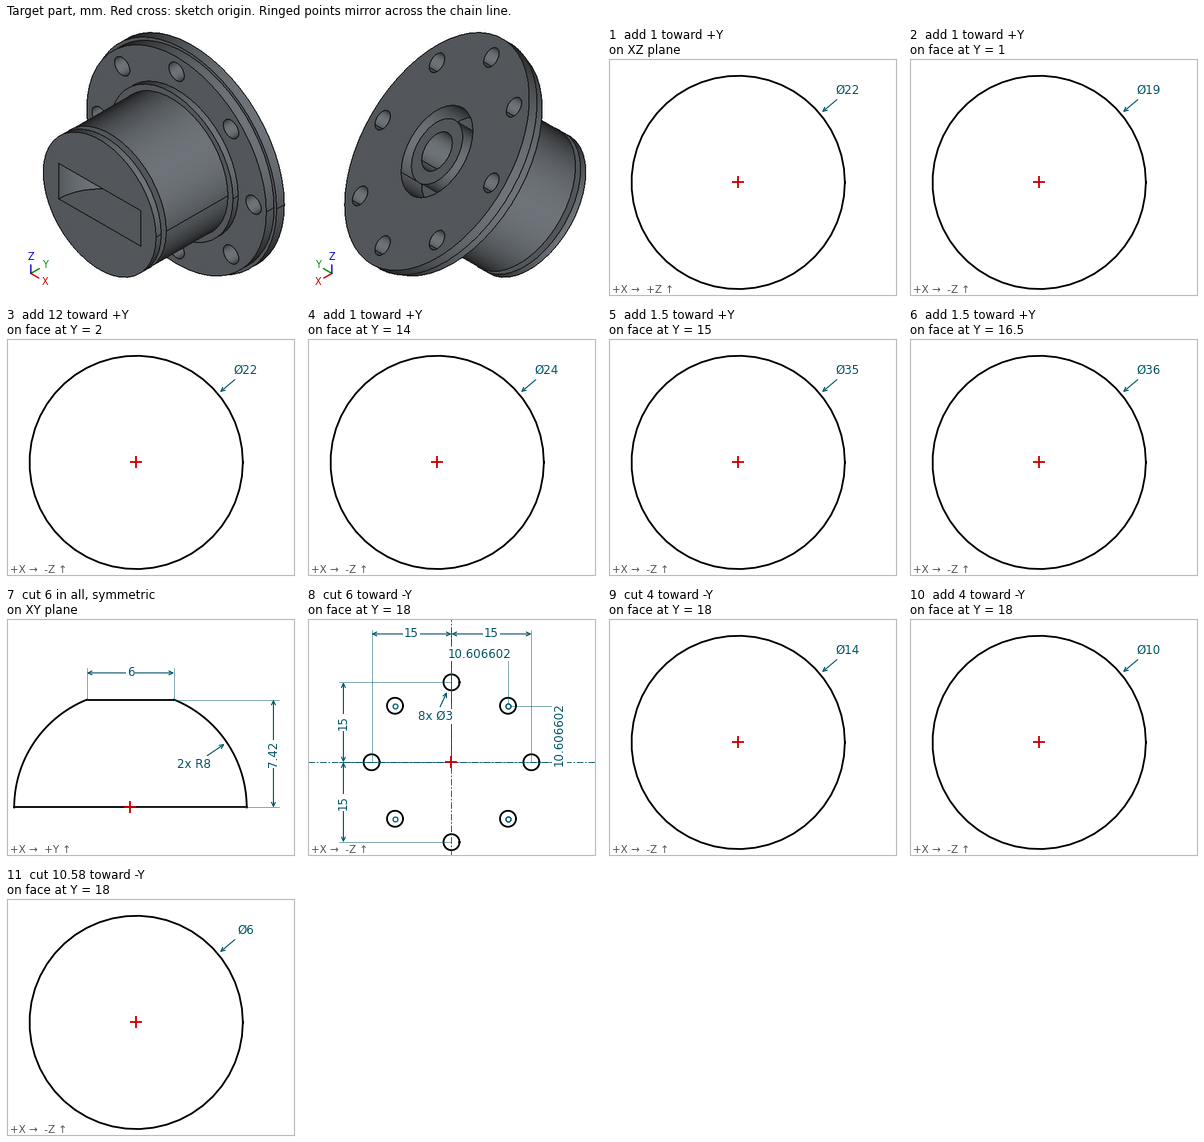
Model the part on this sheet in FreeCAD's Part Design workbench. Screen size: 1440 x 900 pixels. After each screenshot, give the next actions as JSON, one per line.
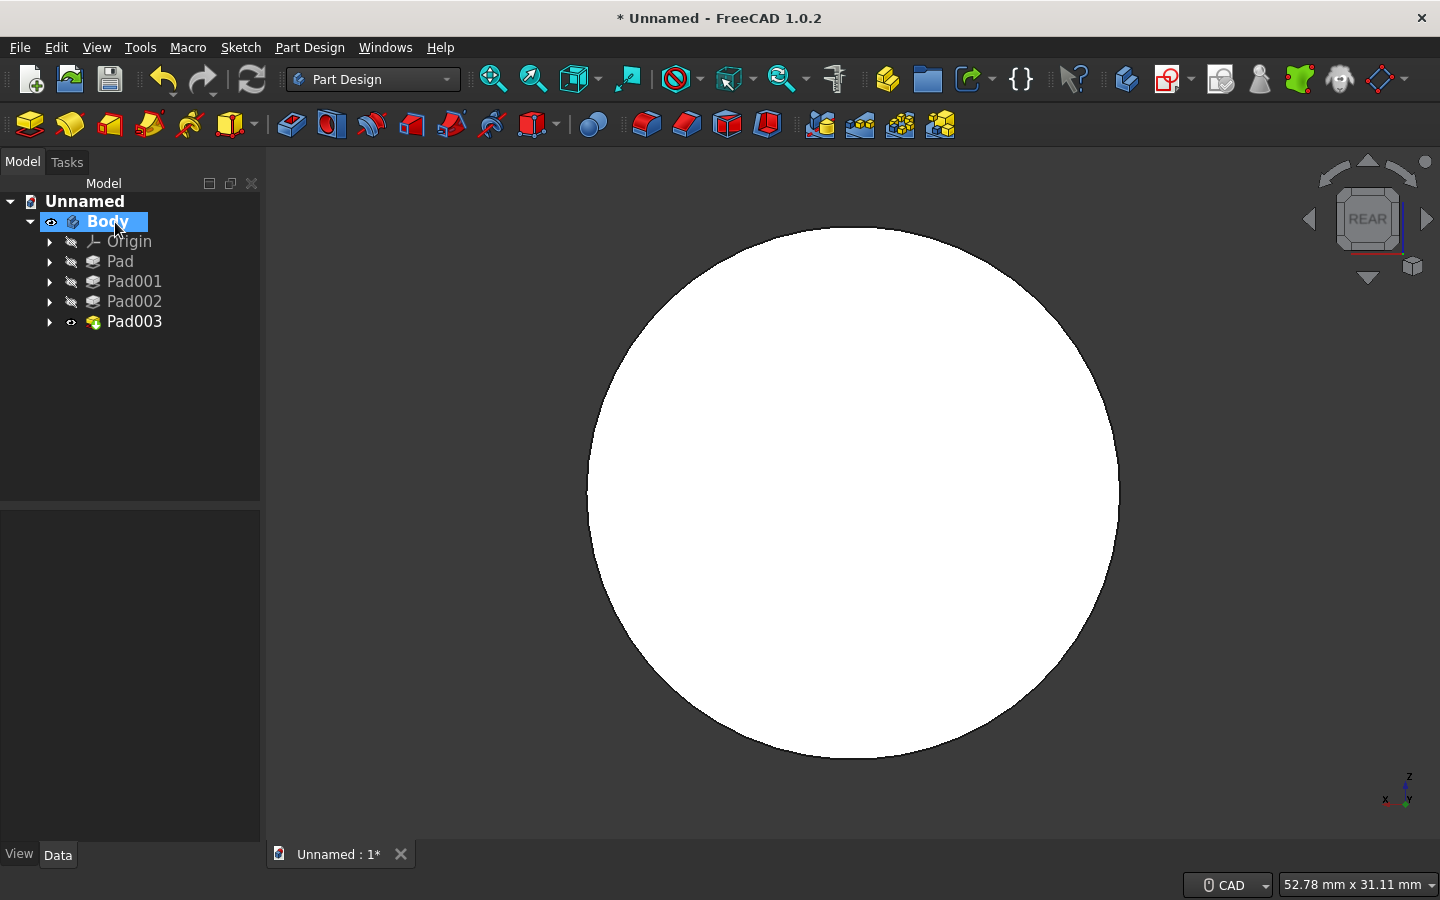
{"action": "left_click", "coordinate": [853, 492]}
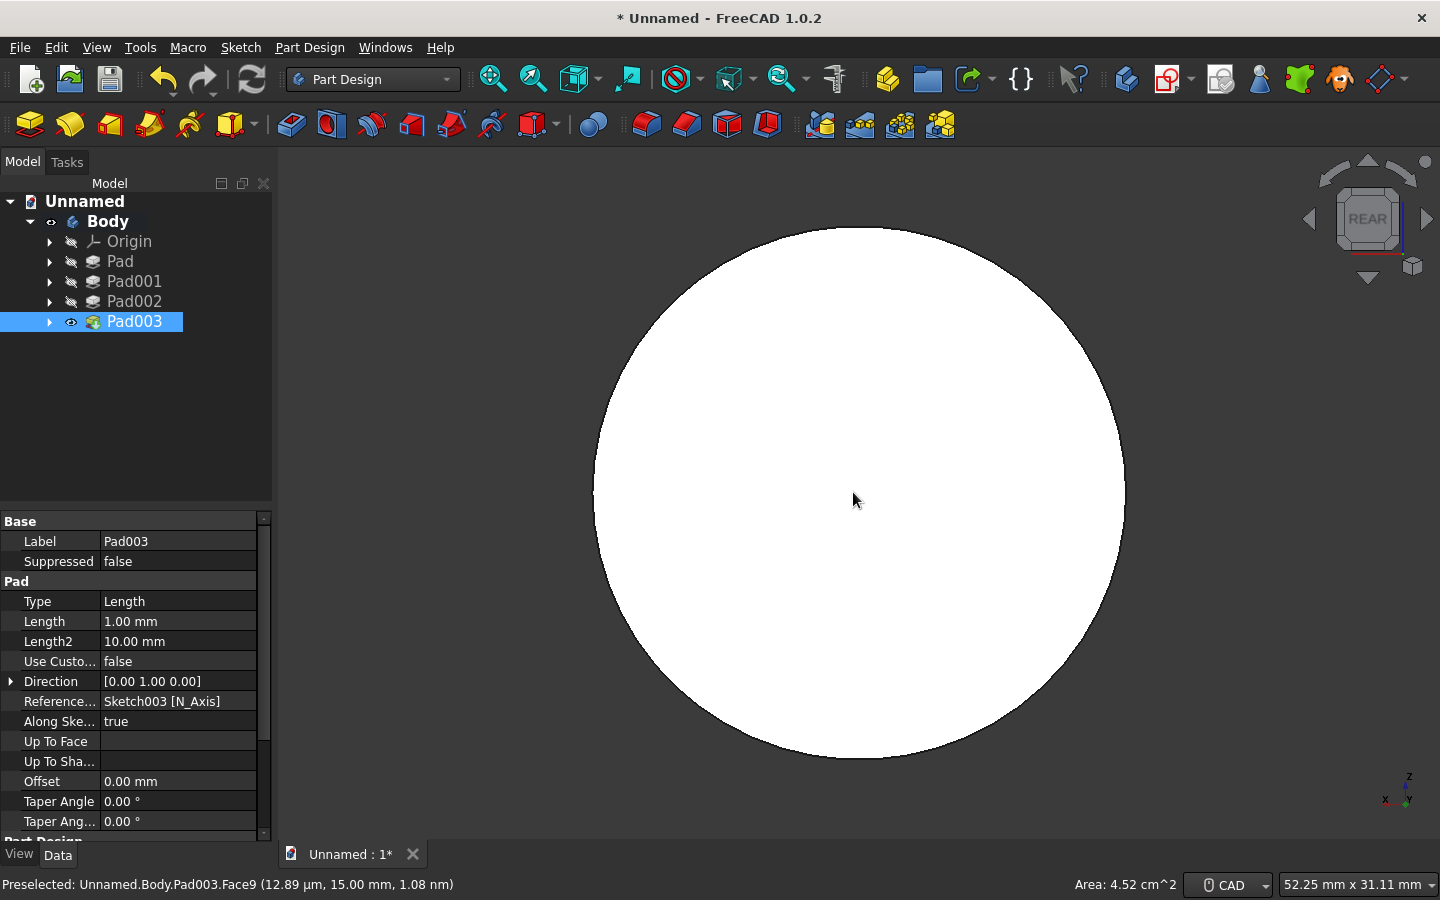
{"action": "left_click", "coordinate": [1168, 80]}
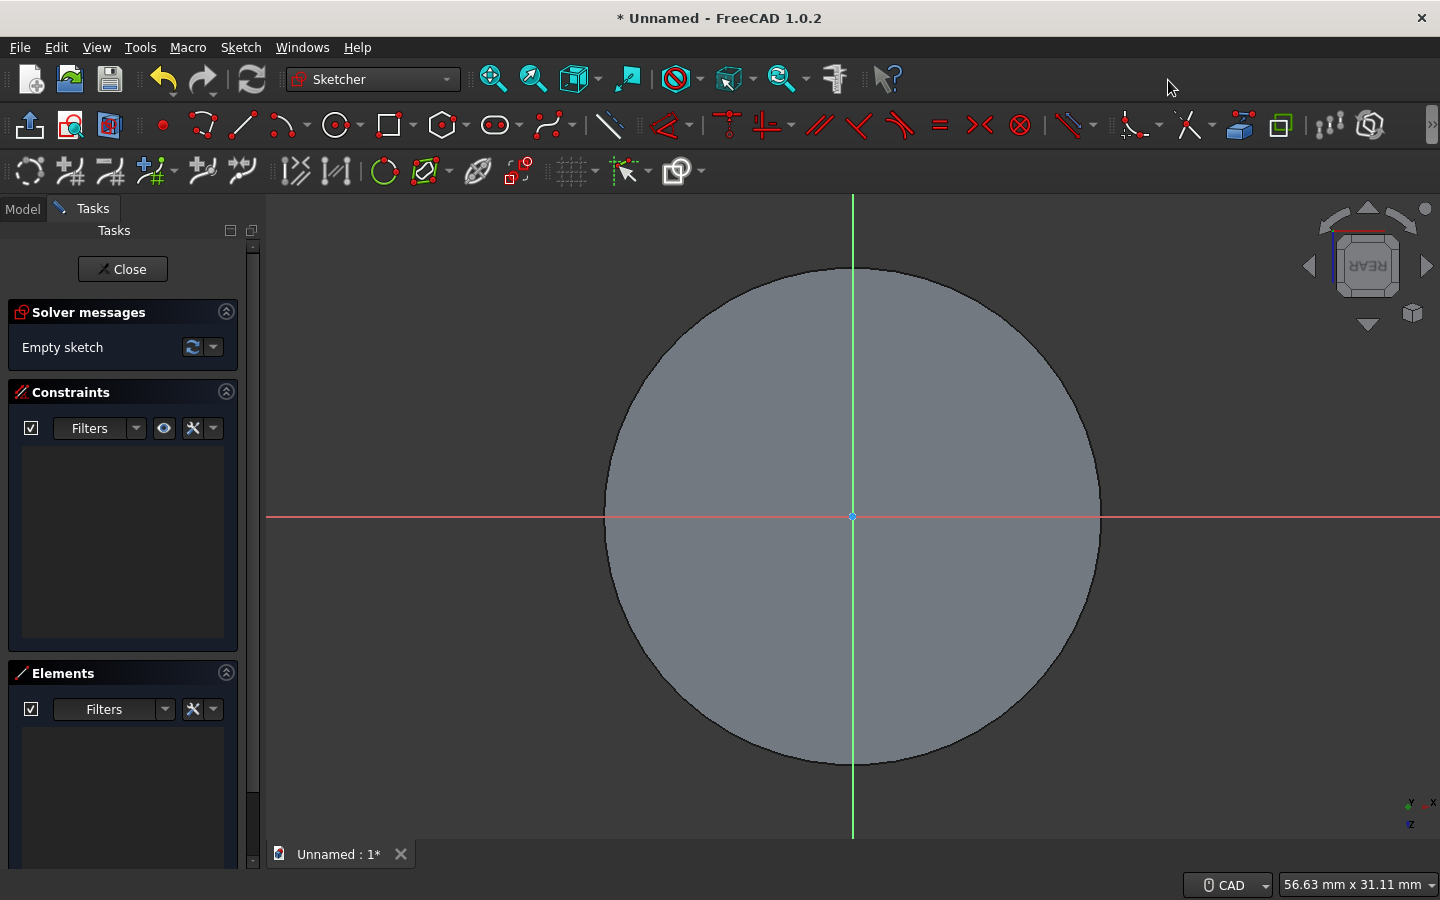
{"action": "scroll", "coordinate": [702, 517], "scroll_direction": "down", "scroll_amount": 3}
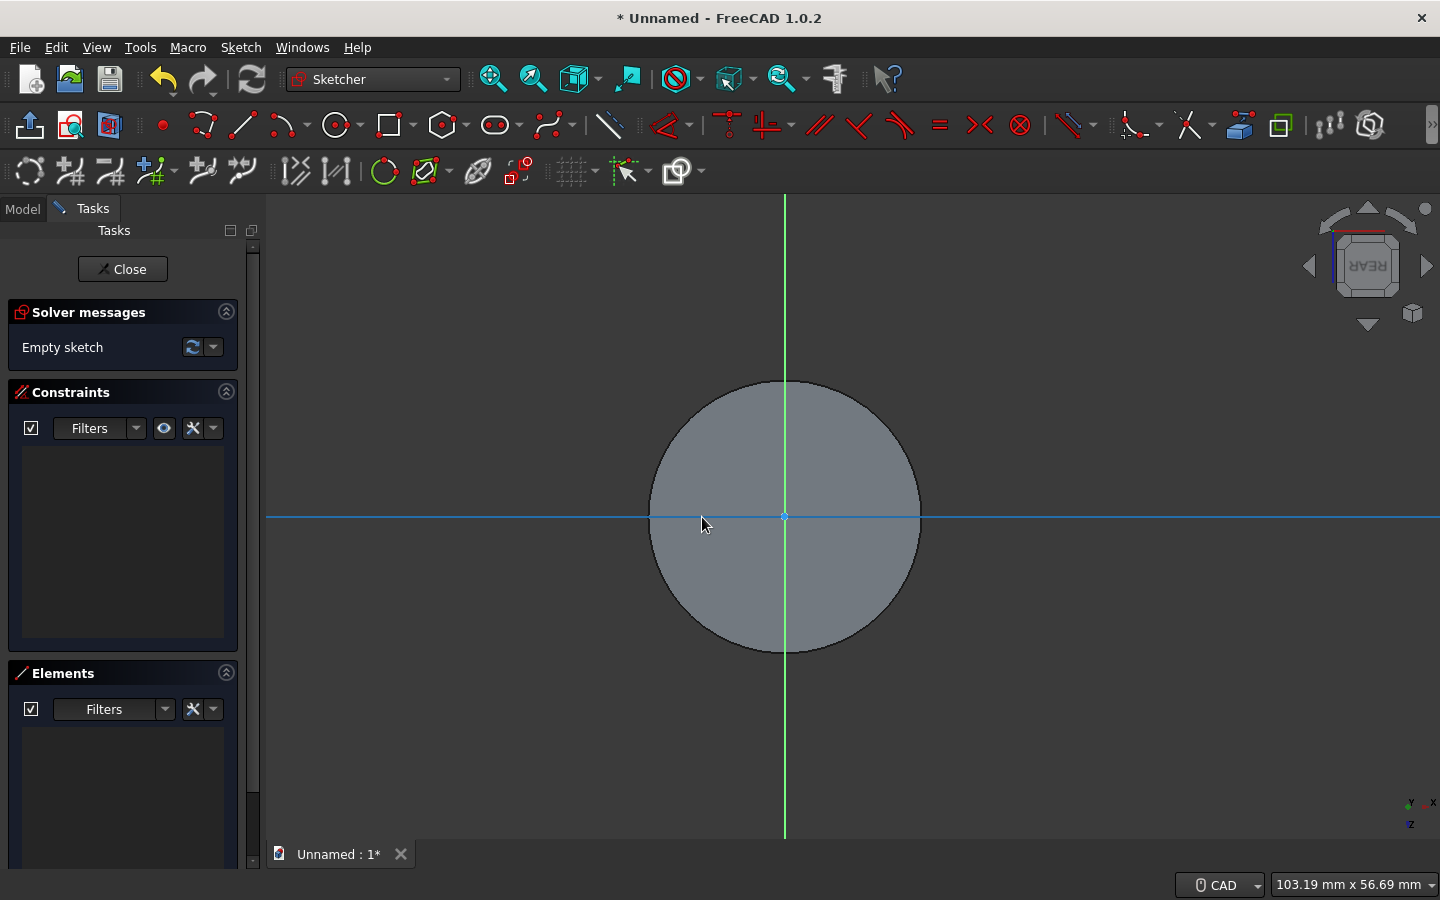
{"action": "left_click", "coordinate": [336, 126]}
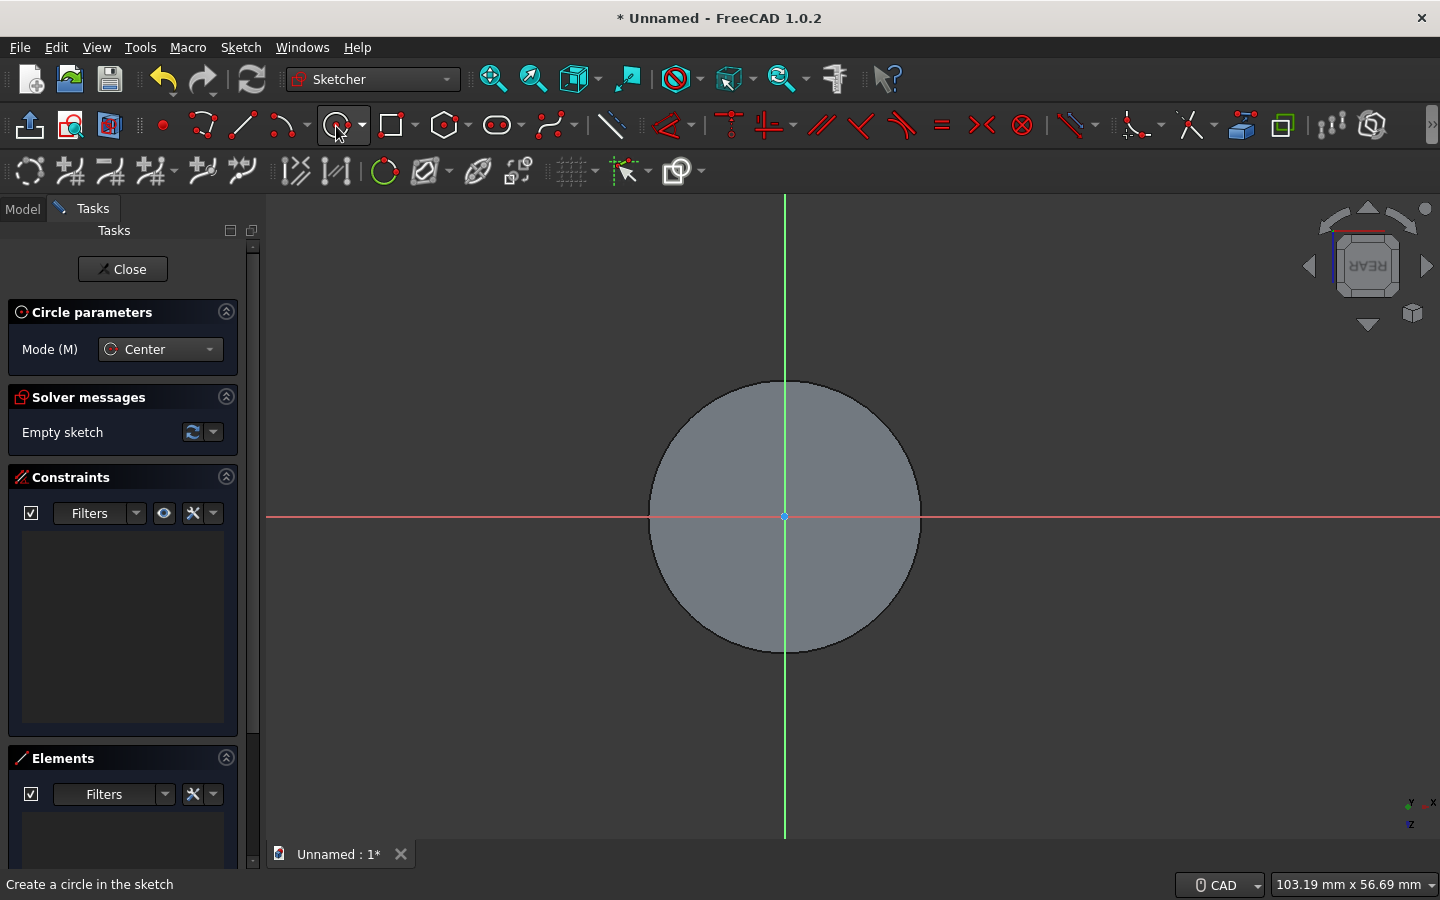
{"action": "left_click", "coordinate": [785, 517]}
{"action": "mouse_move", "coordinate": [926, 376]}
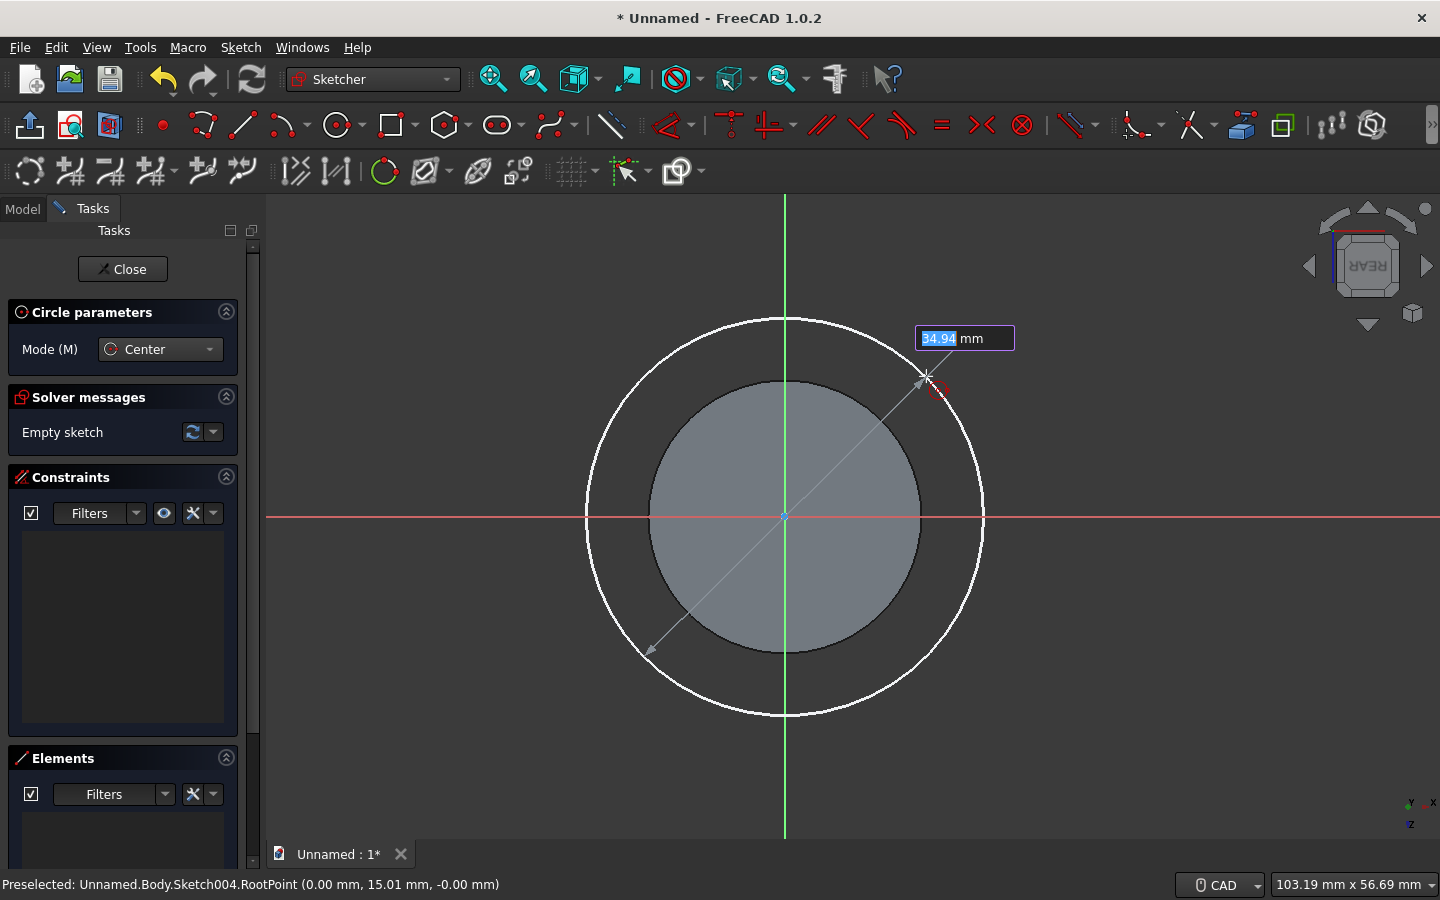
{"action": "type", "text": "35"}
{"action": "key", "text": "Return"}
{"action": "key", "text": "Escape"}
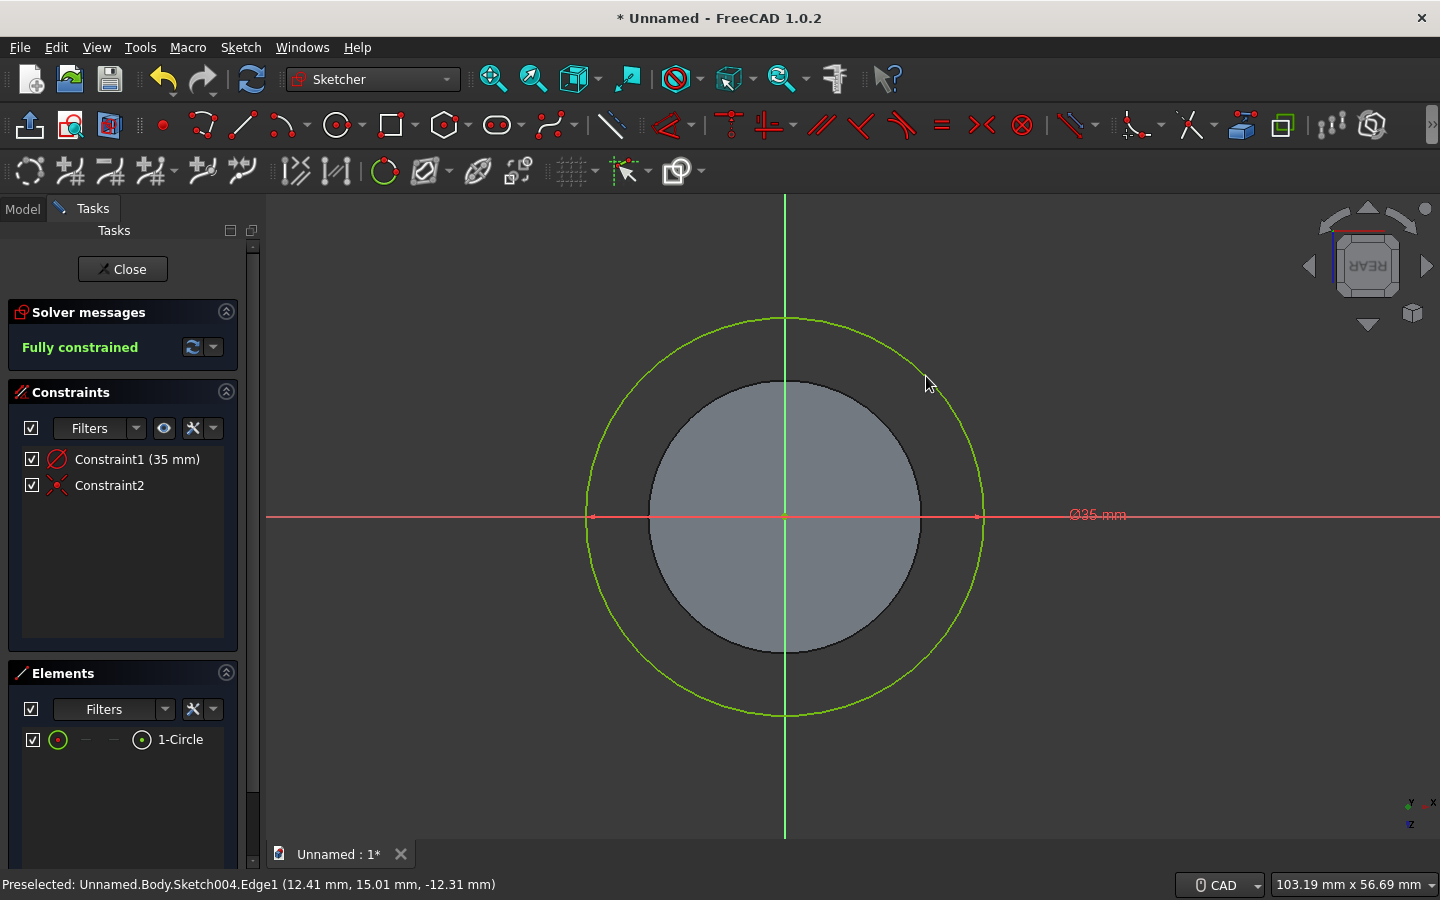
{"action": "left_click", "coordinate": [123, 269]}